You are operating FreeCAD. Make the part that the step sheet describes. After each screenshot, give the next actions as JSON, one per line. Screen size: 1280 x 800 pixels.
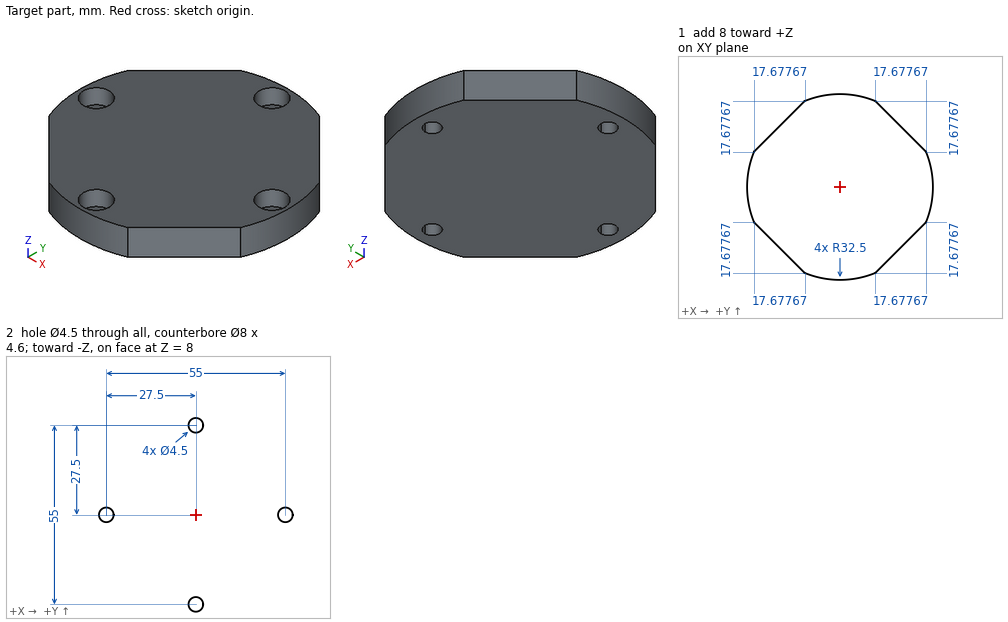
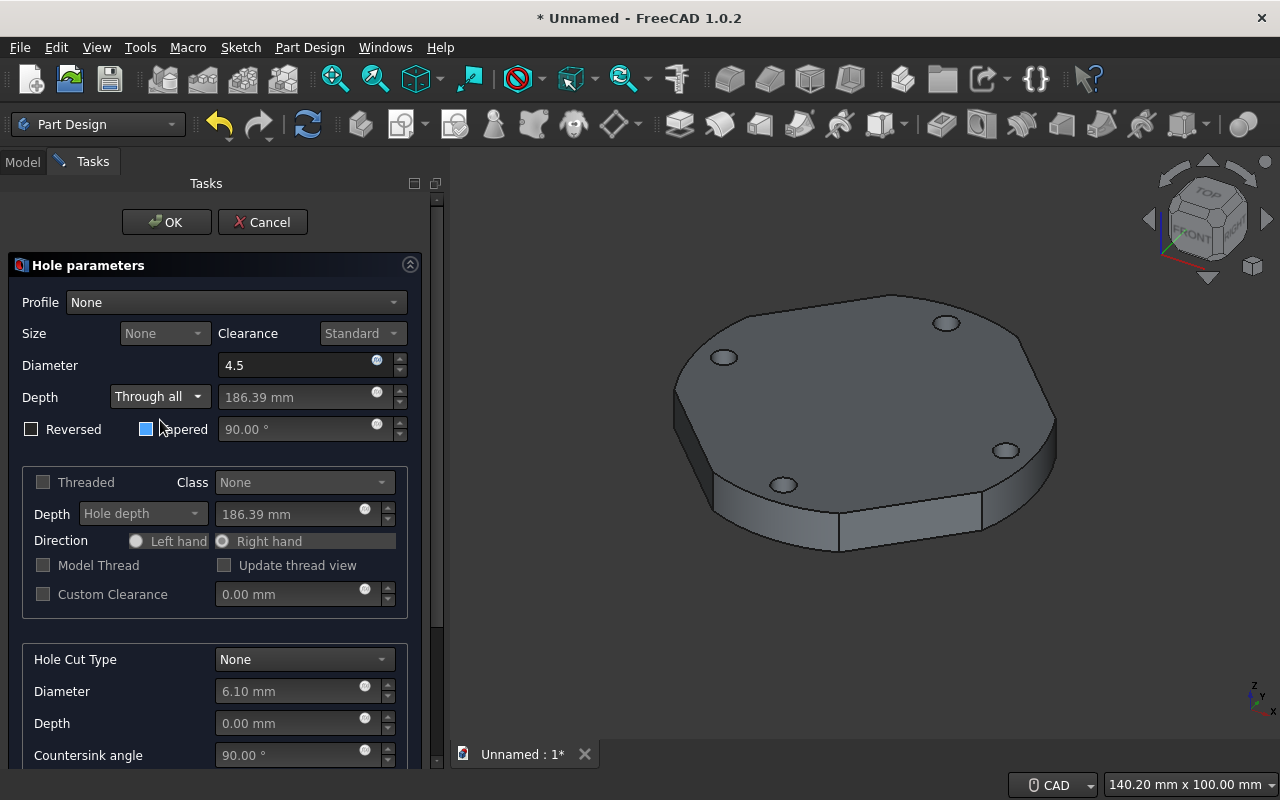
{"action": "left_click", "coordinate": [306, 660]}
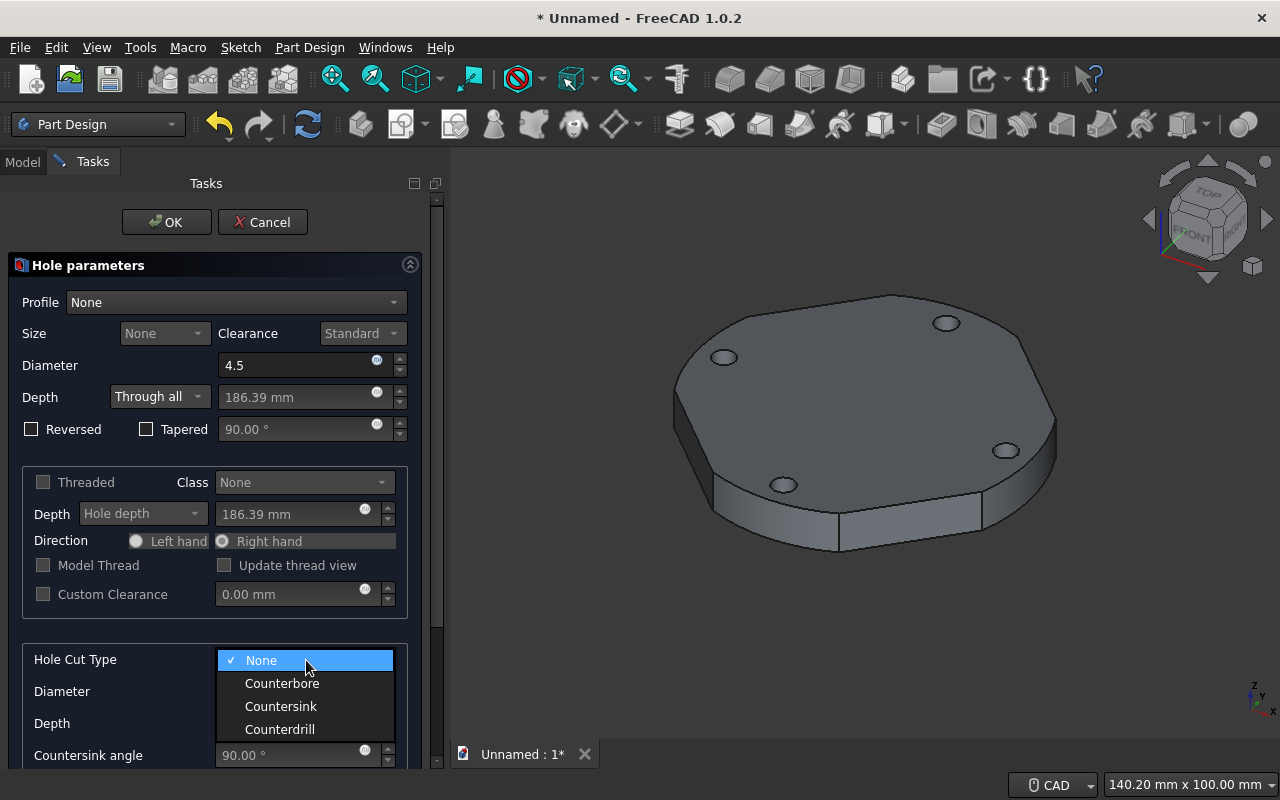
{"action": "left_click", "coordinate": [304, 684]}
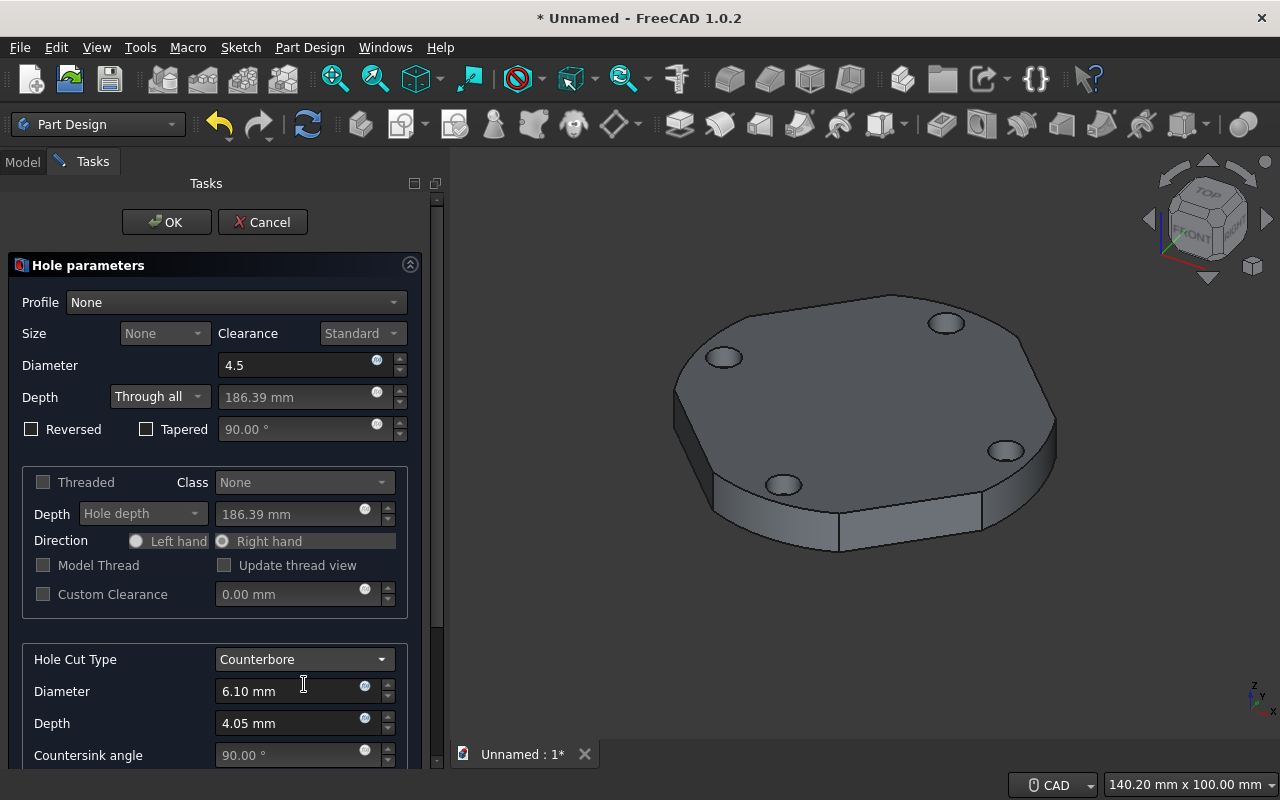
{"action": "triple_click", "coordinate": [298, 691]}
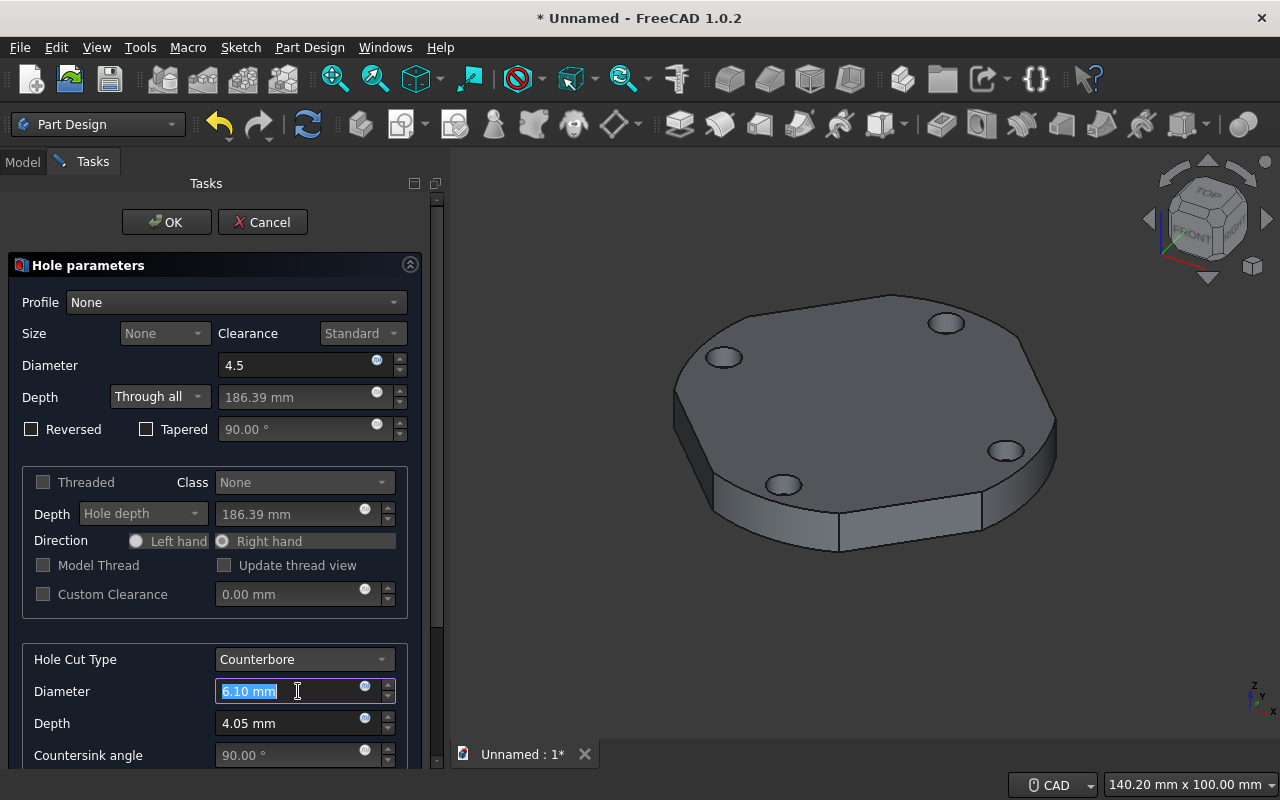
{"action": "type", "text": "8"}
{"action": "key", "text": "Tab"}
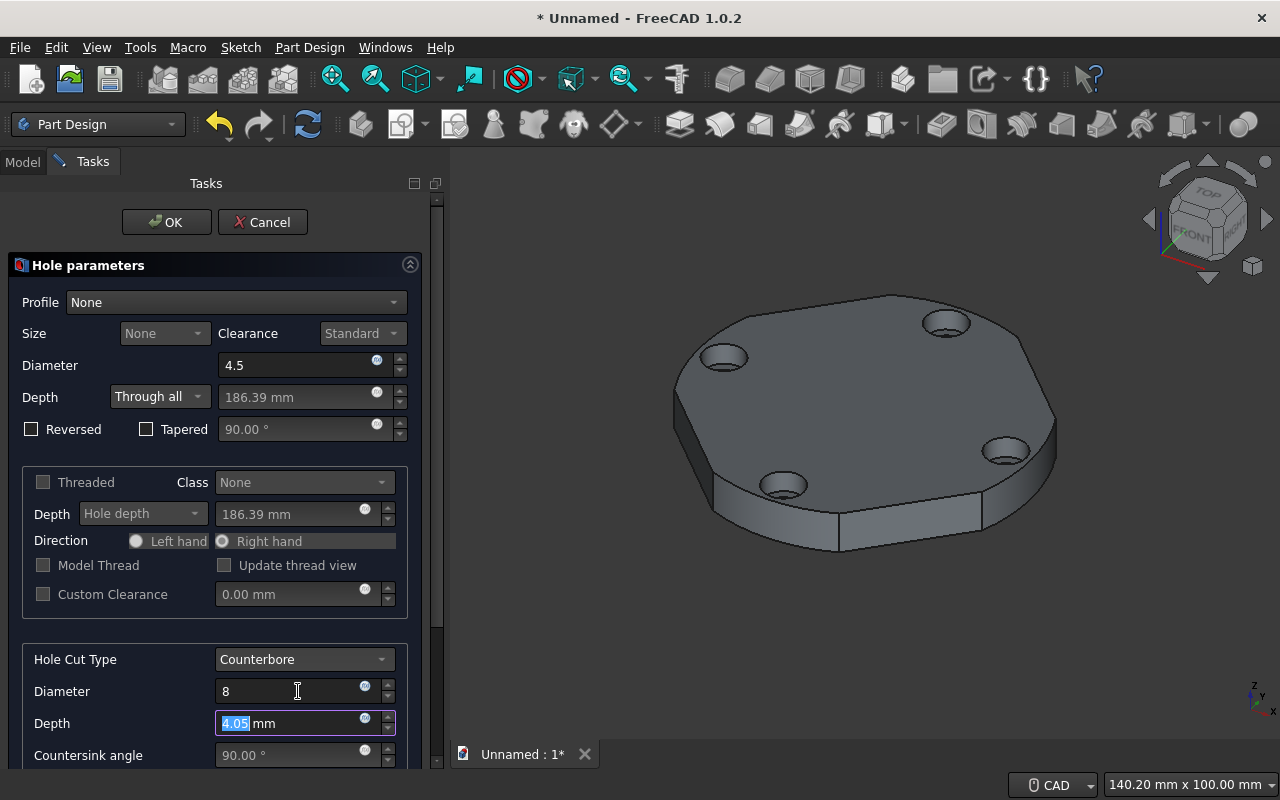
{"action": "type", "text": "4.6"}
{"action": "key", "text": "Tab"}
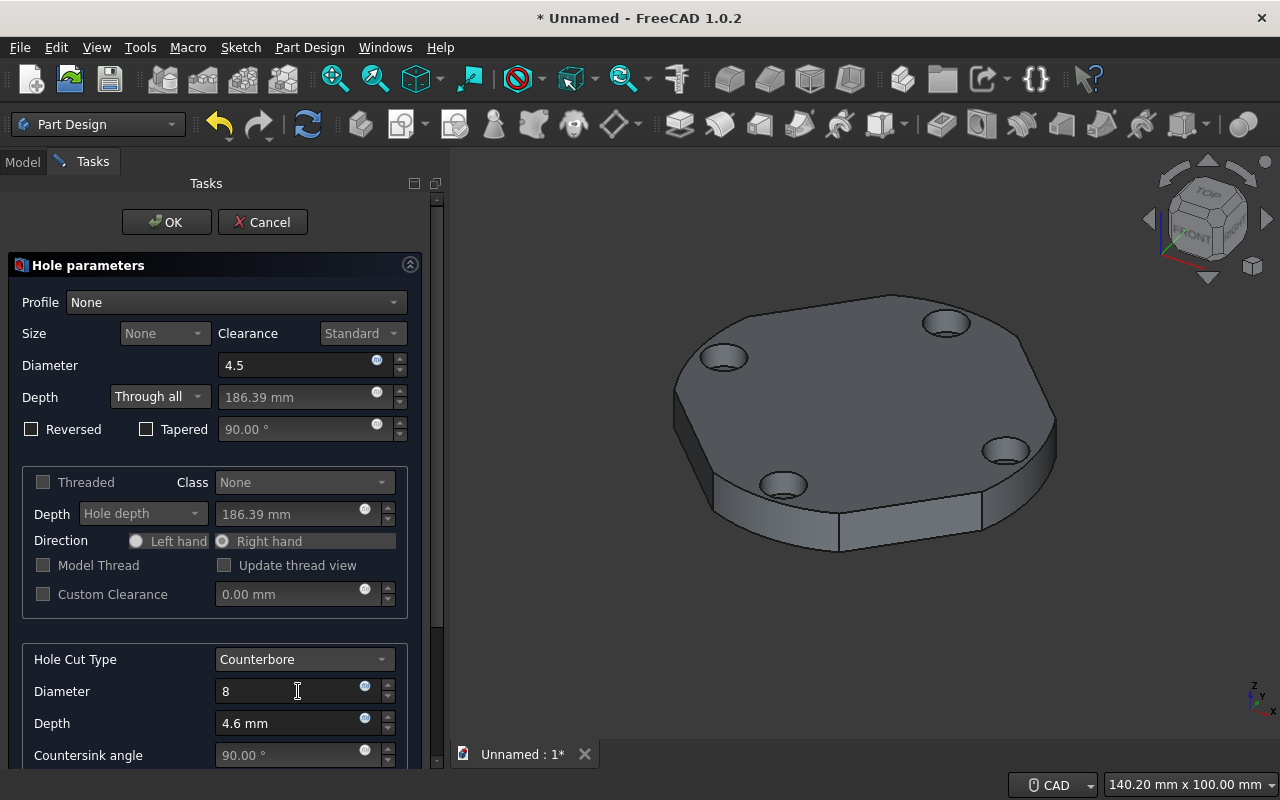
{"action": "left_click", "coordinate": [167, 222]}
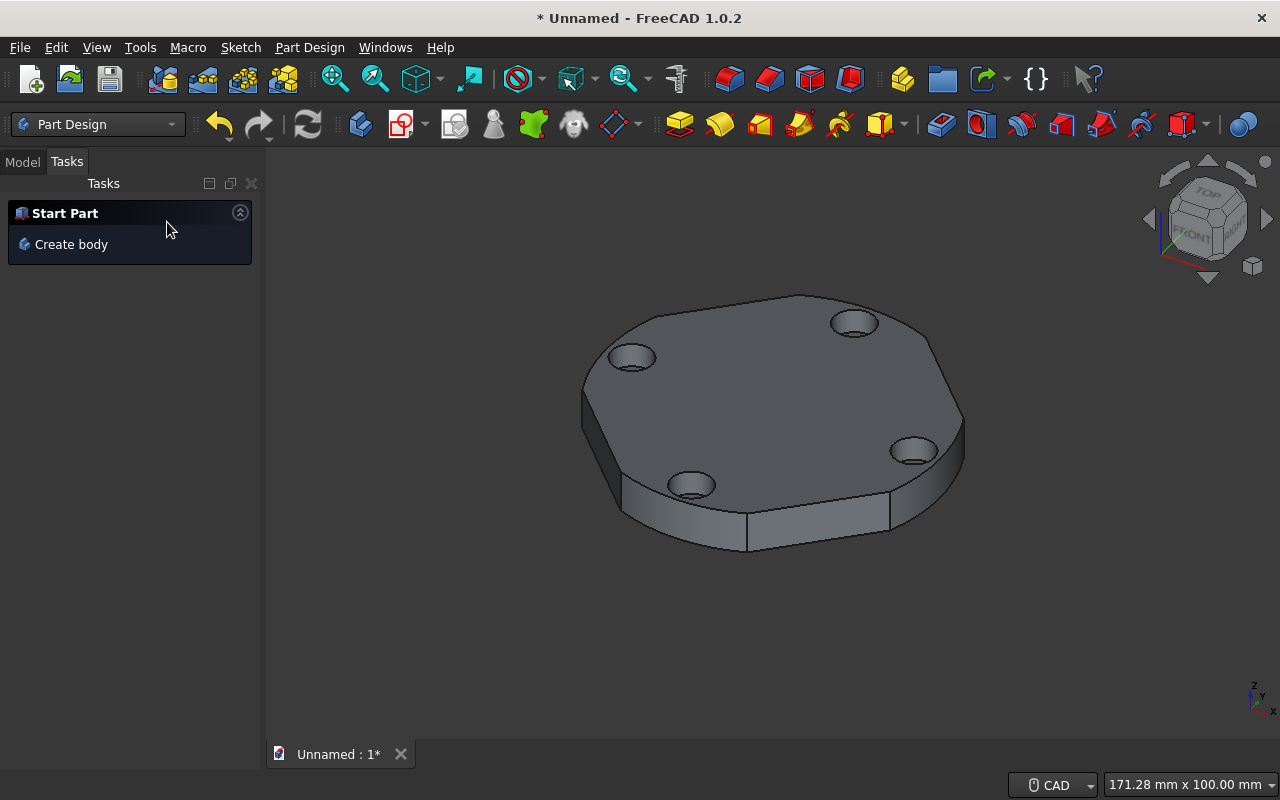
{"action": "key", "text": "0"}